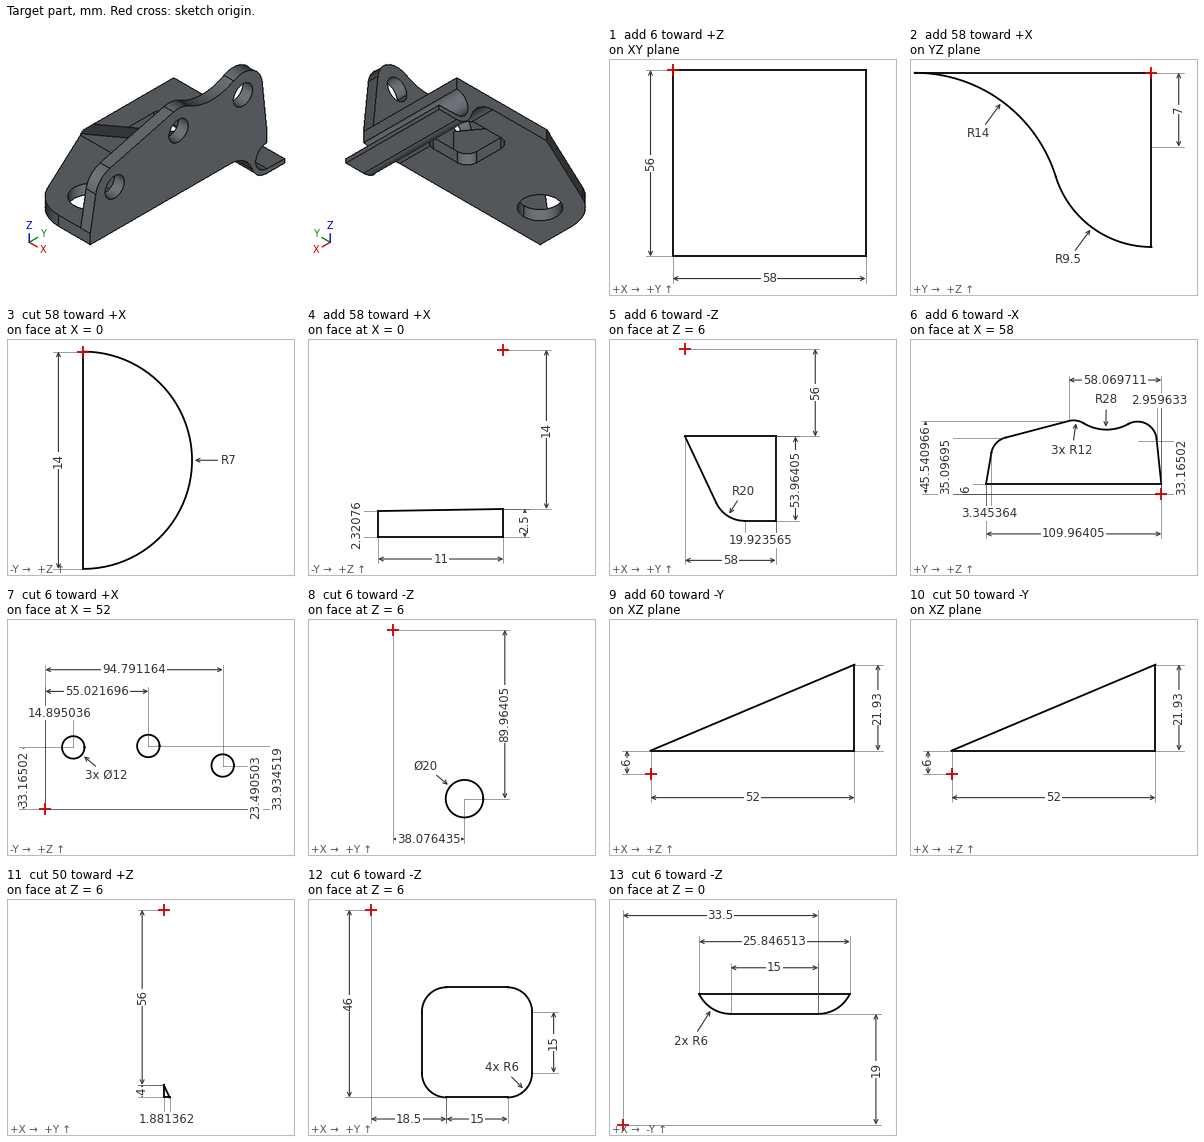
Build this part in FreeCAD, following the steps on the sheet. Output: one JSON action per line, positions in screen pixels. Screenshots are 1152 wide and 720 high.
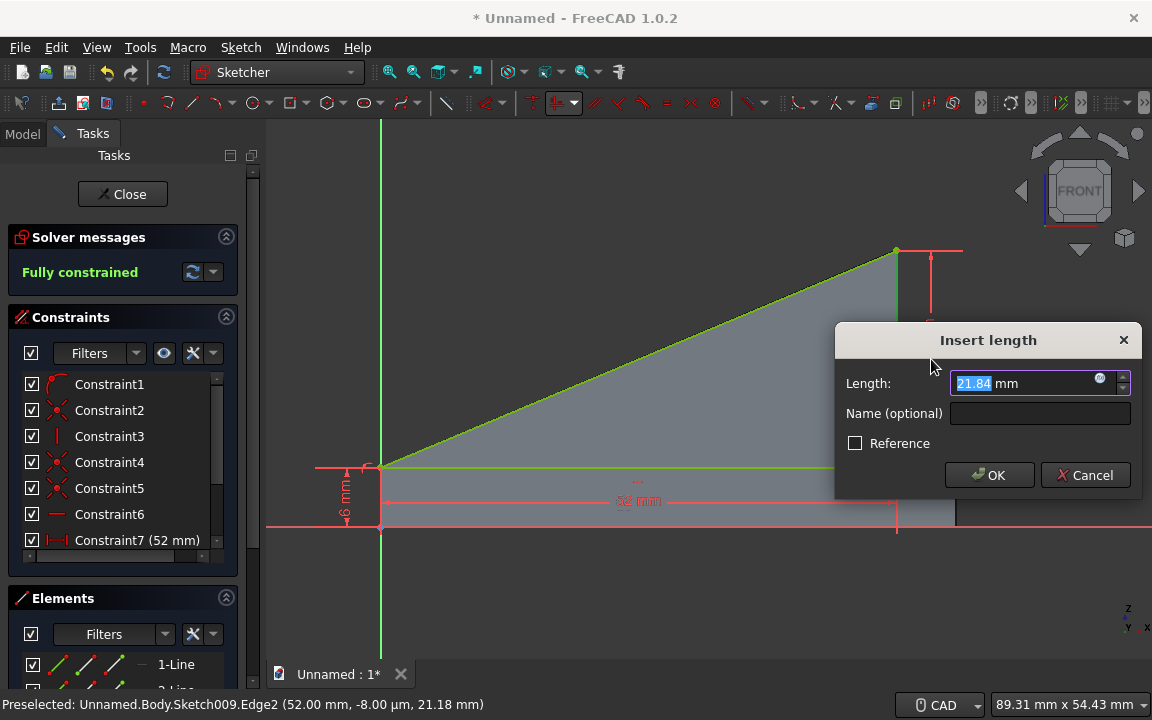
{"action": "type", "text": "21.93"}
{"action": "key", "text": "Return"}
{"action": "key", "text": "Escape"}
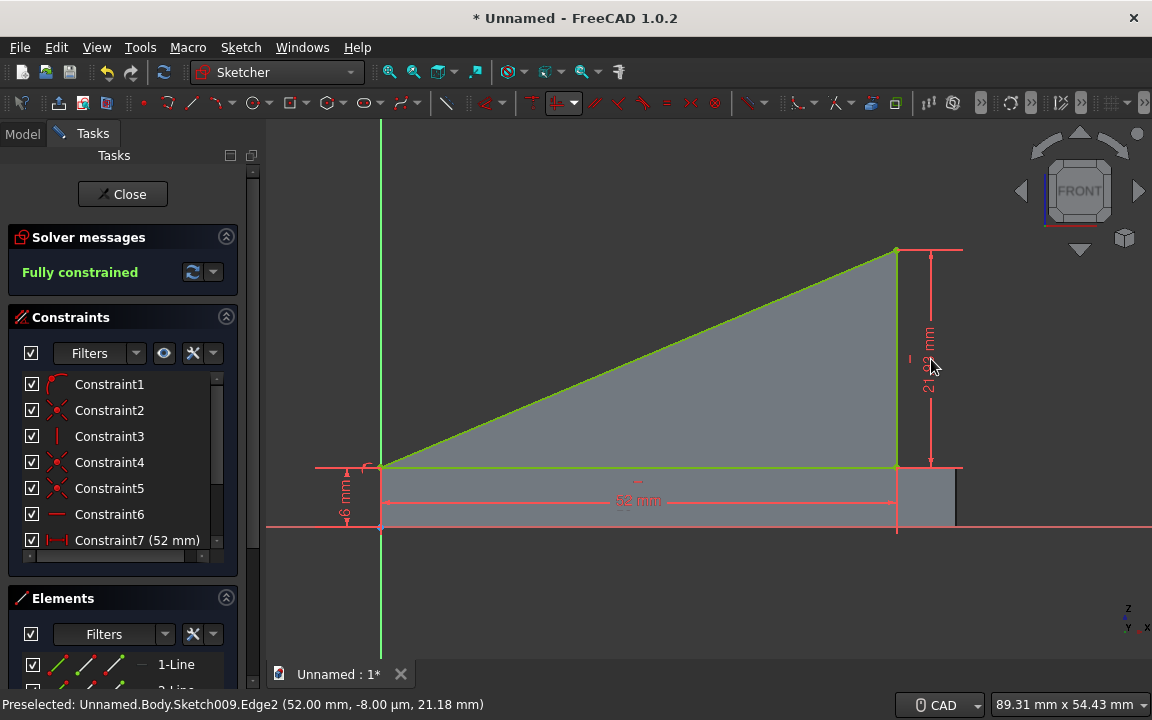
{"action": "left_click", "coordinate": [123, 194]}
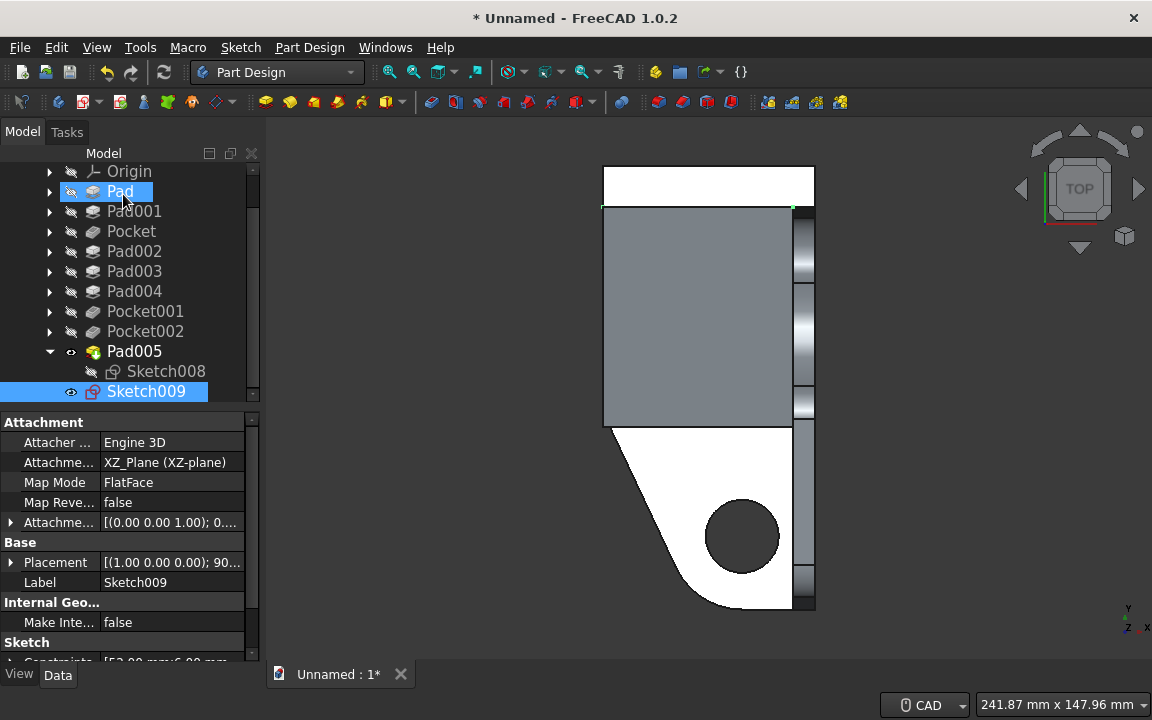
{"action": "left_click", "coordinate": [432, 102]}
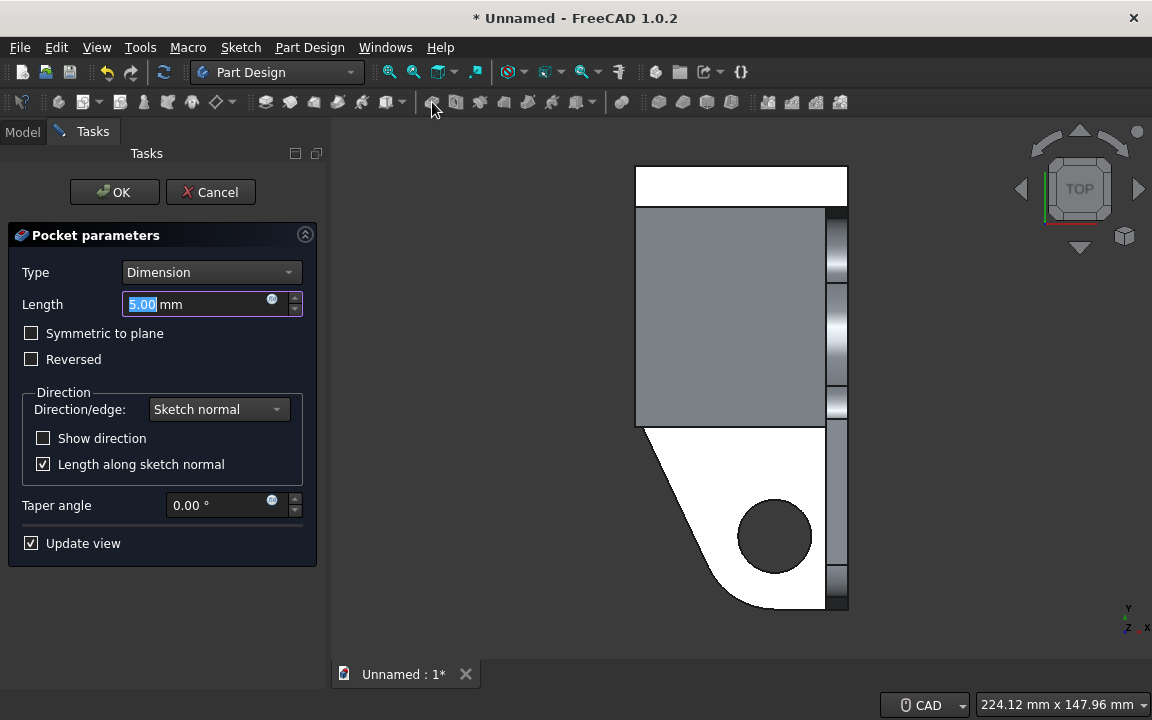
{"action": "type", "text": "50"}
{"action": "key", "text": "Tab"}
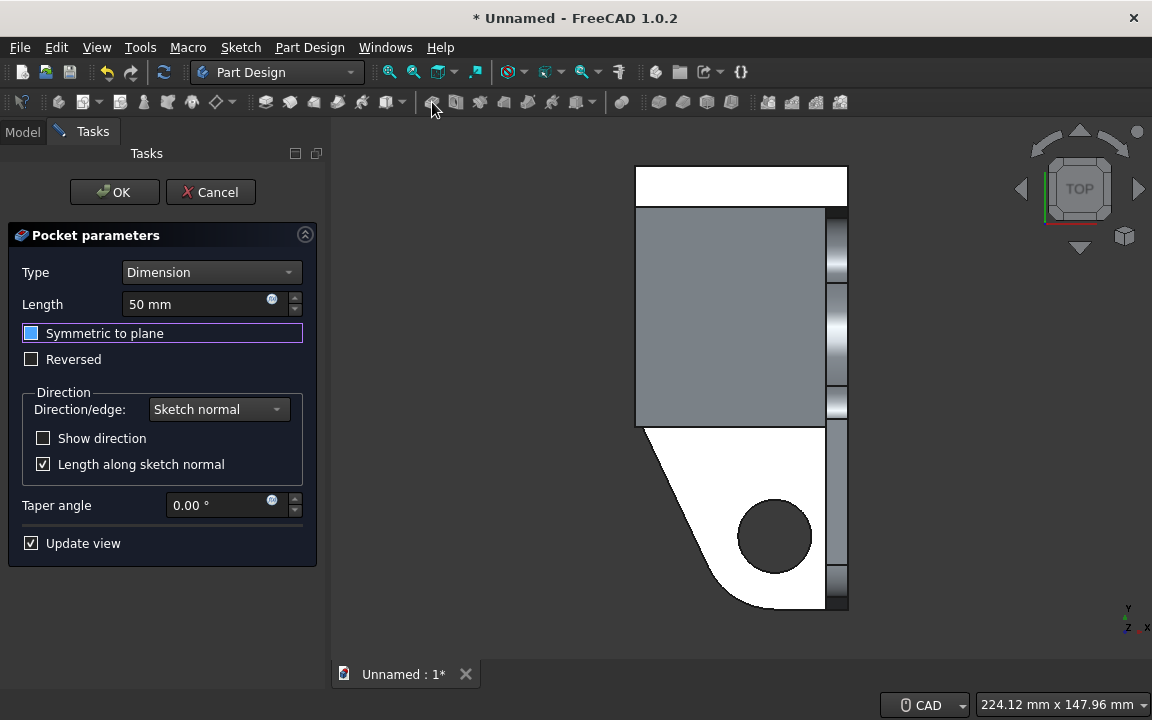
{"action": "left_click", "coordinate": [30, 359]}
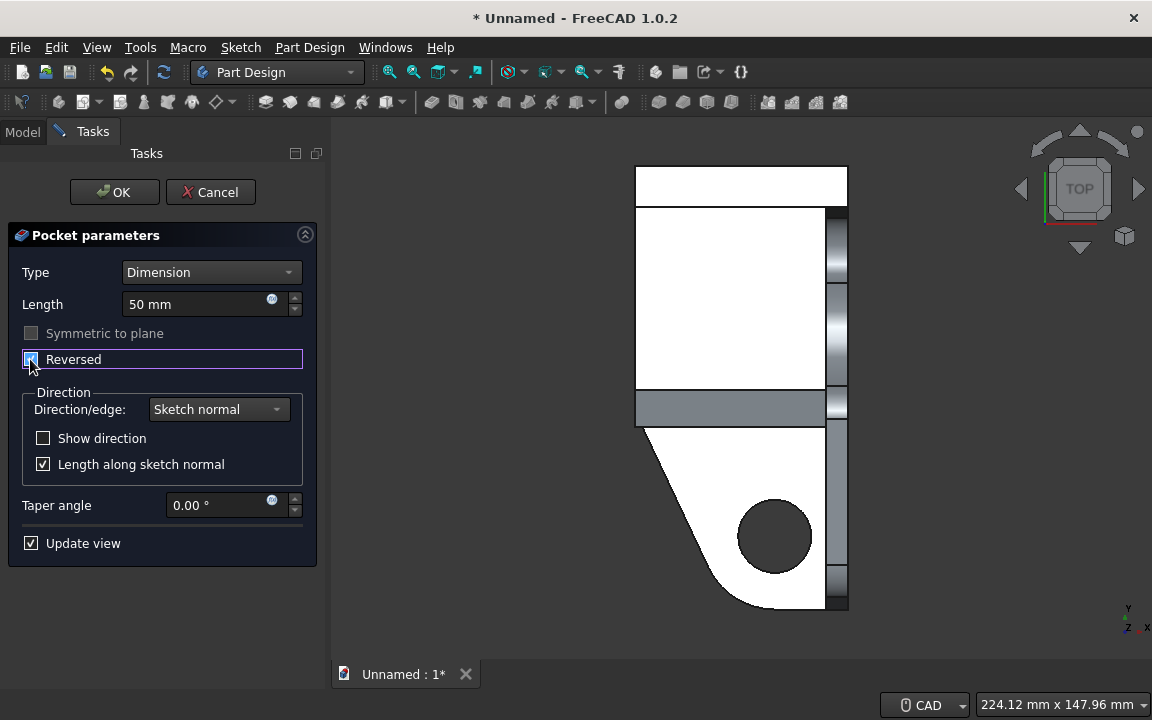
{"action": "left_click", "coordinate": [115, 192]}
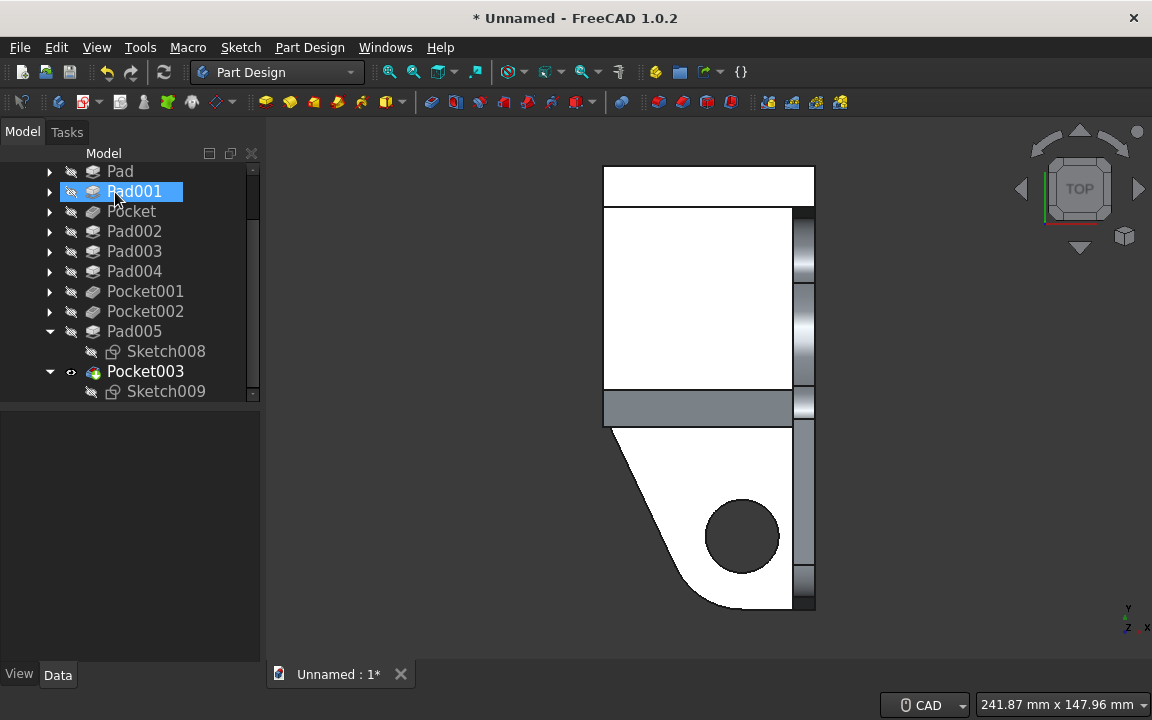
{"action": "left_click", "coordinate": [698, 297]}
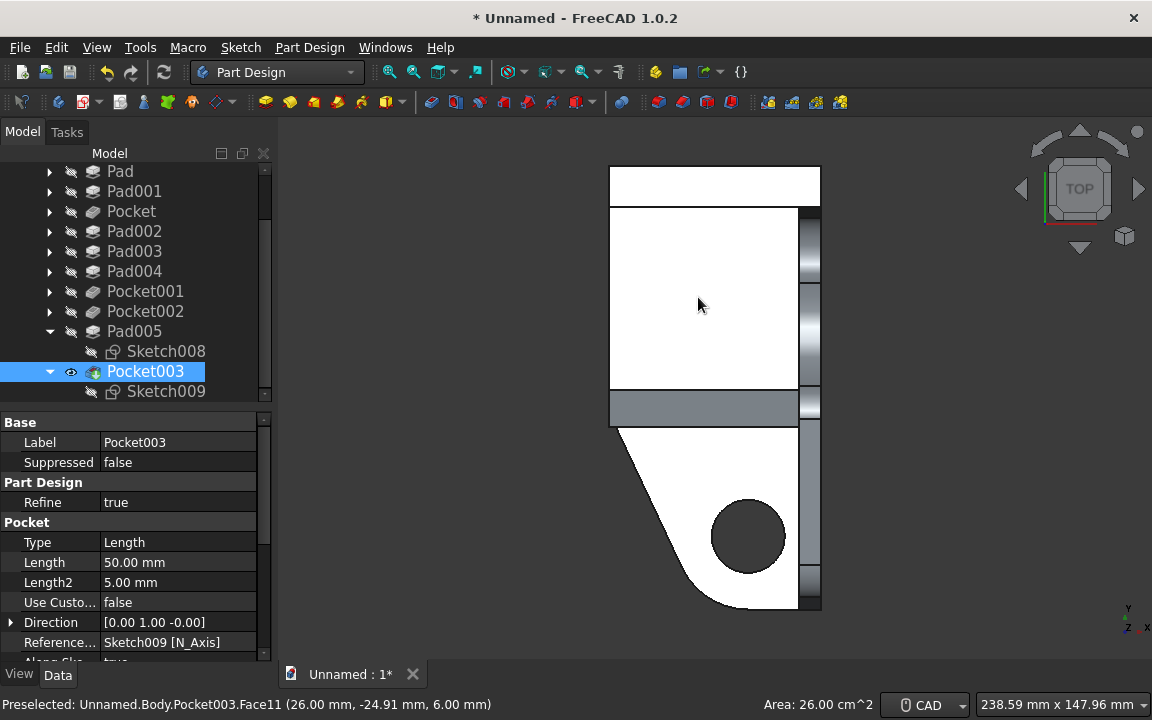
{"action": "left_click", "coordinate": [84, 102]}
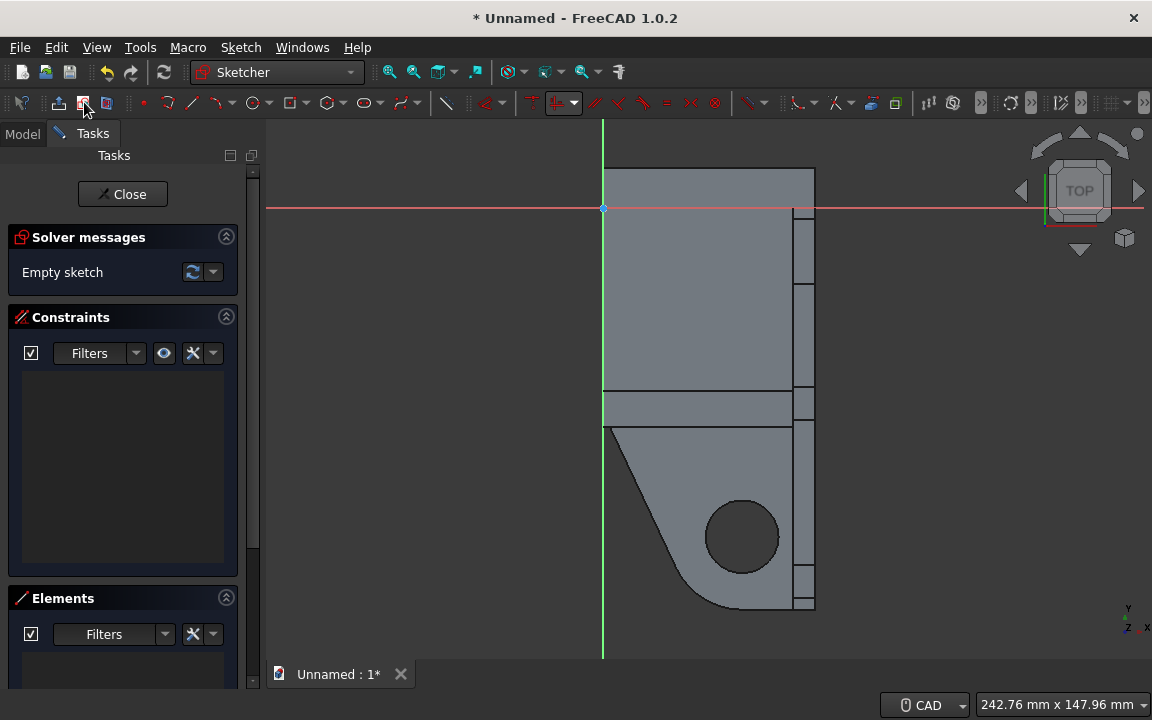
{"action": "left_click", "coordinate": [108, 104]}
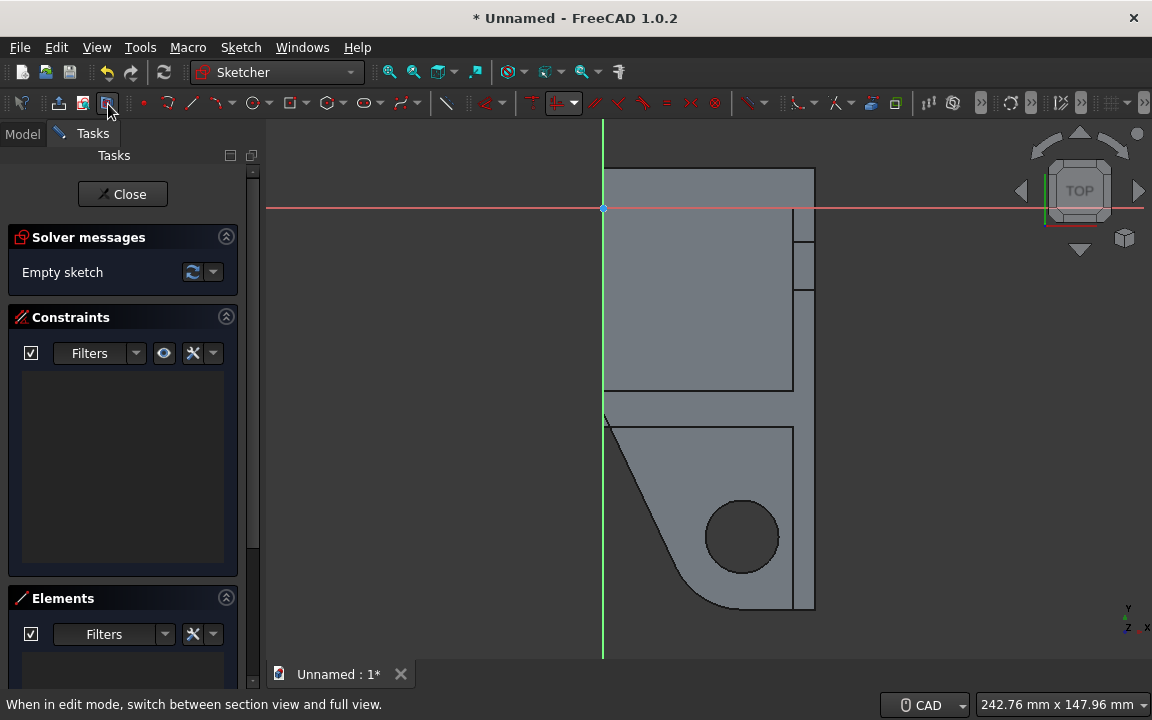
{"action": "scroll", "coordinate": [605, 422], "scroll_direction": "up", "scroll_amount": 15}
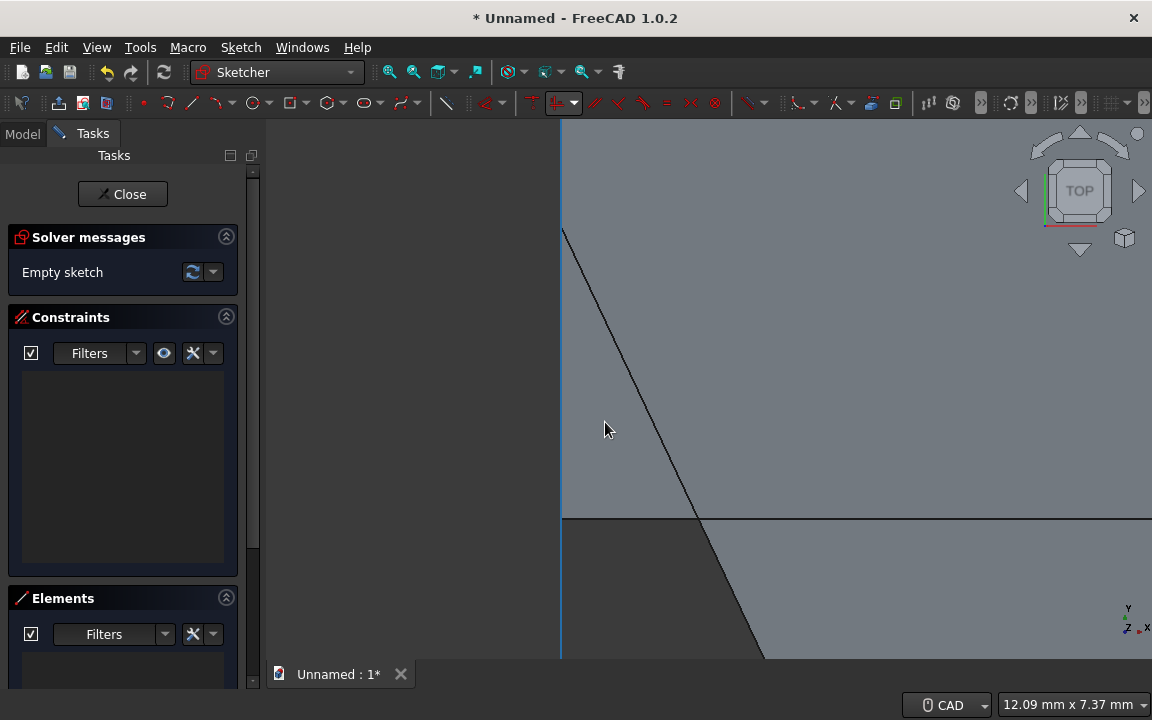
{"action": "left_click", "coordinate": [168, 104]}